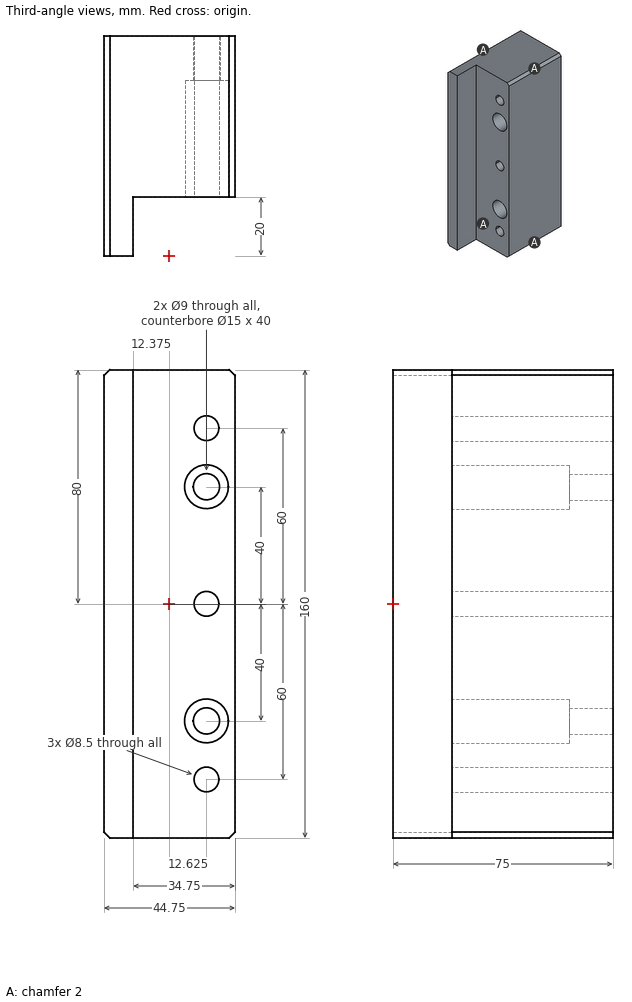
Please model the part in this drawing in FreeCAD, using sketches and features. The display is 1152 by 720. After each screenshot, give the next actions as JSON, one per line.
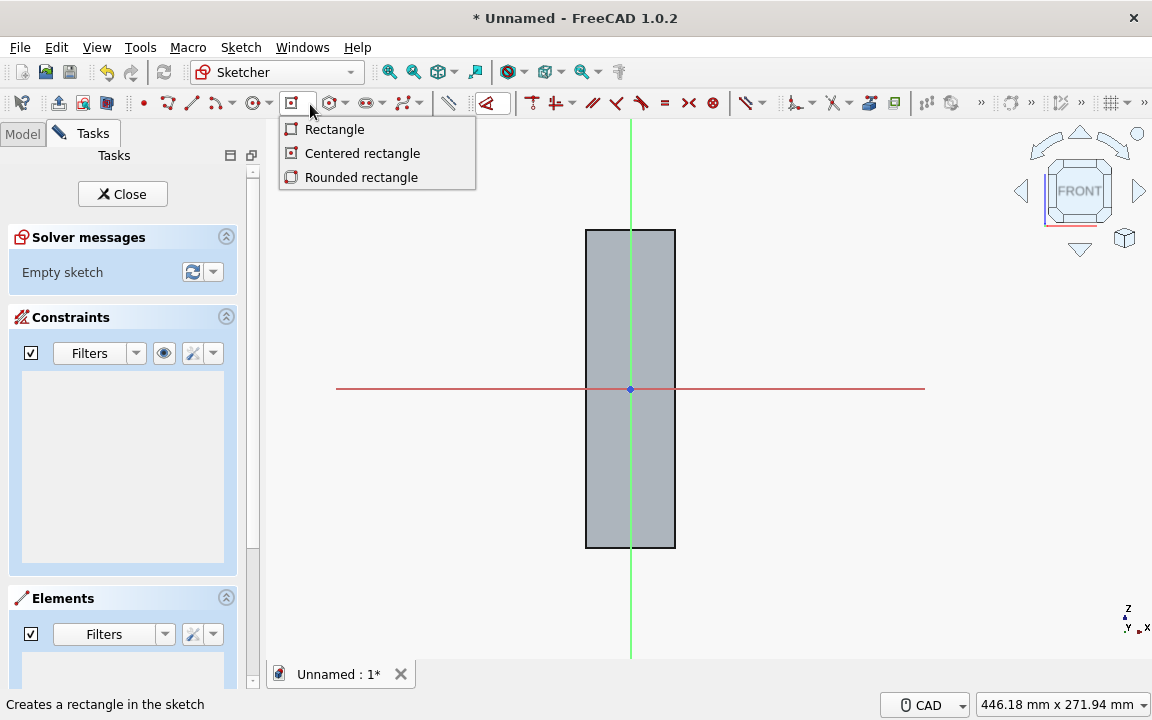
{"action": "left_click", "coordinate": [378, 129]}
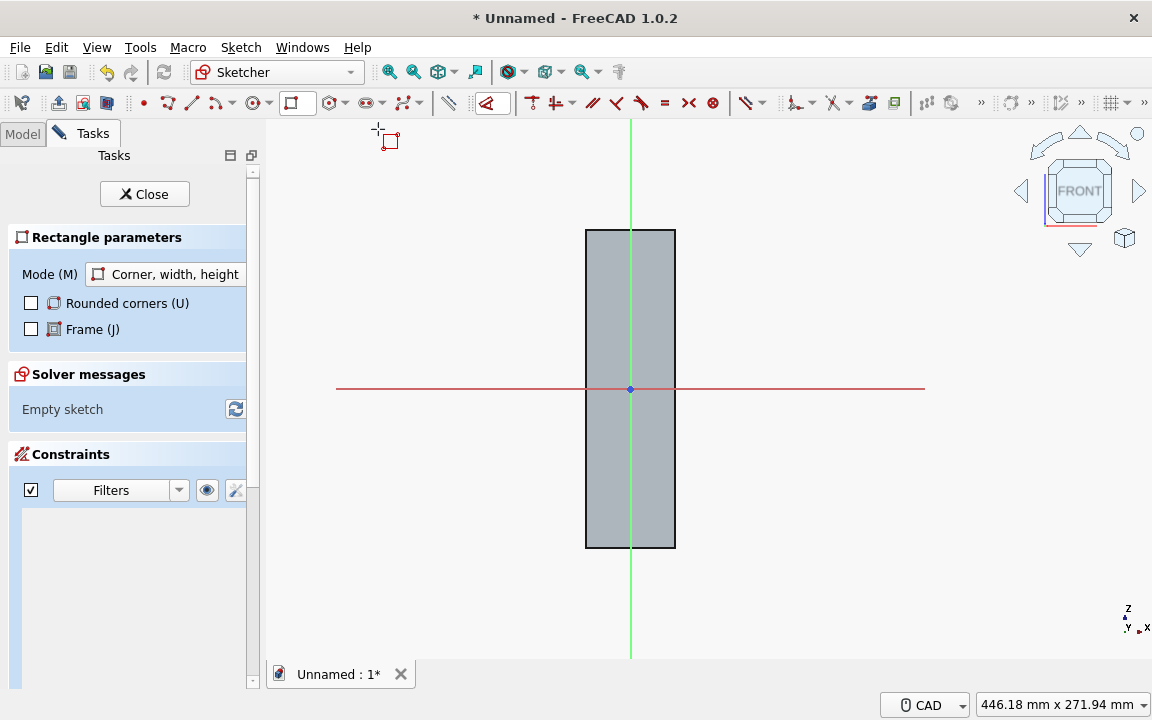
{"action": "left_click", "coordinate": [606, 230]}
{"action": "left_click", "coordinate": [675, 548]}
{"action": "key", "text": "Escape"}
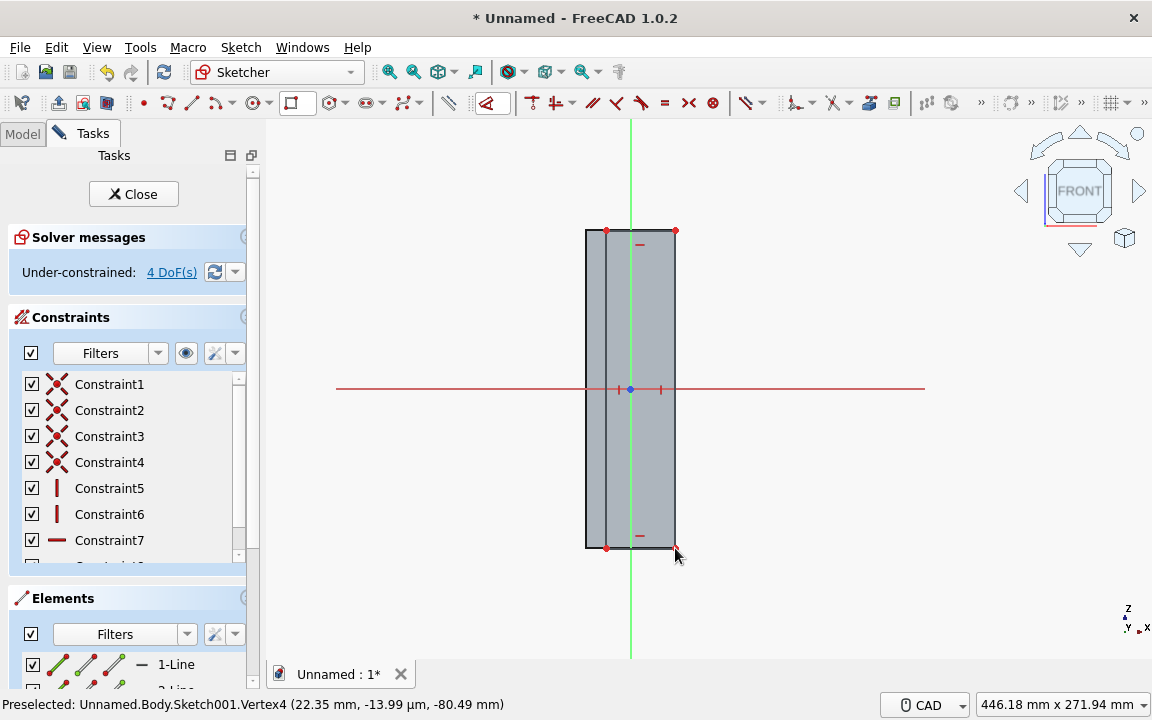
{"action": "key", "text": "d"}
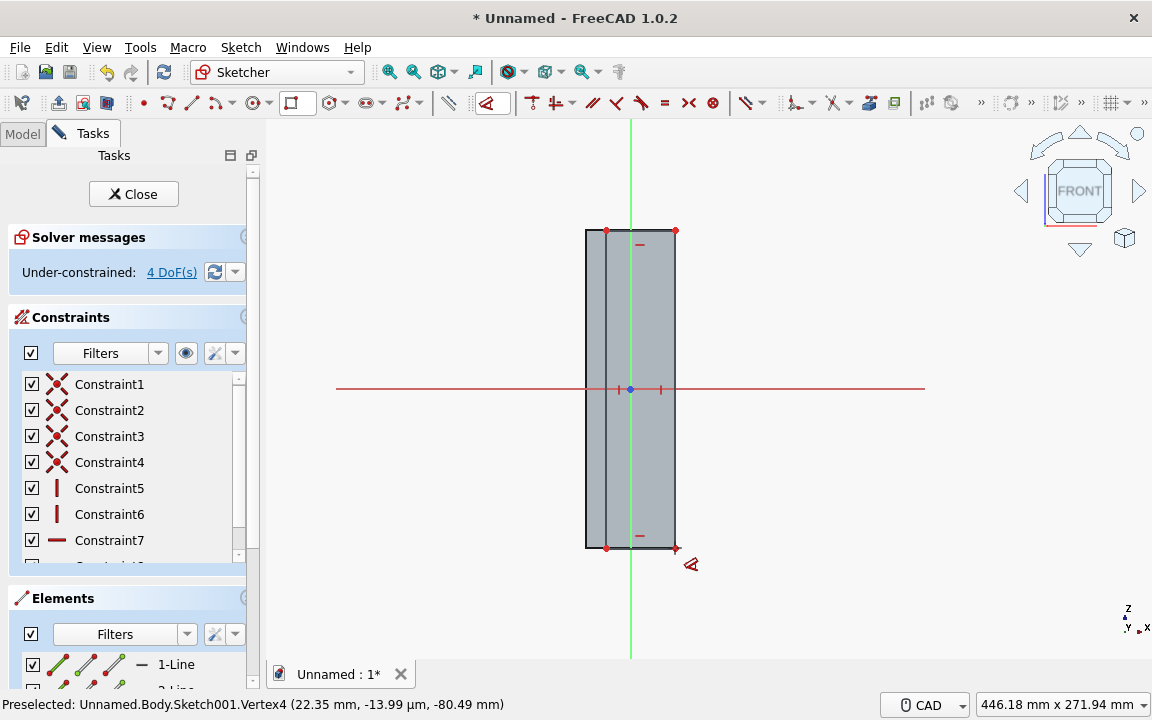
{"action": "left_click", "coordinate": [606, 326]}
{"action": "left_click", "coordinate": [572, 317]}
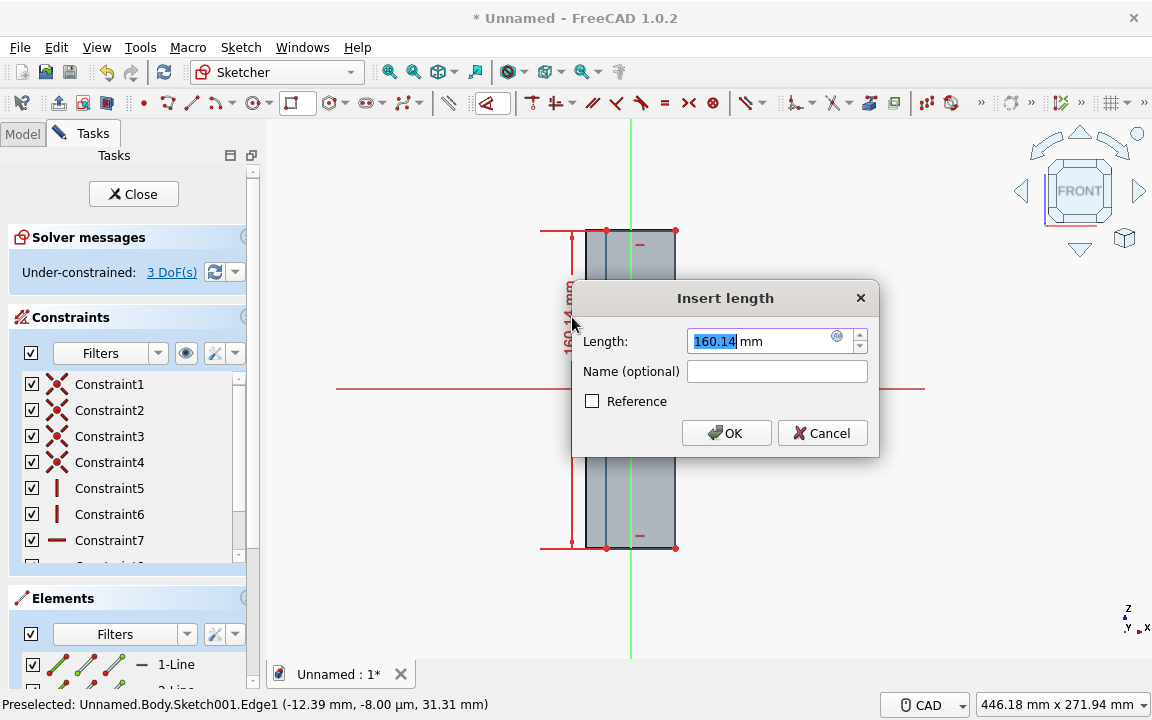
{"action": "type", "text": "160"}
{"action": "key", "text": "Return"}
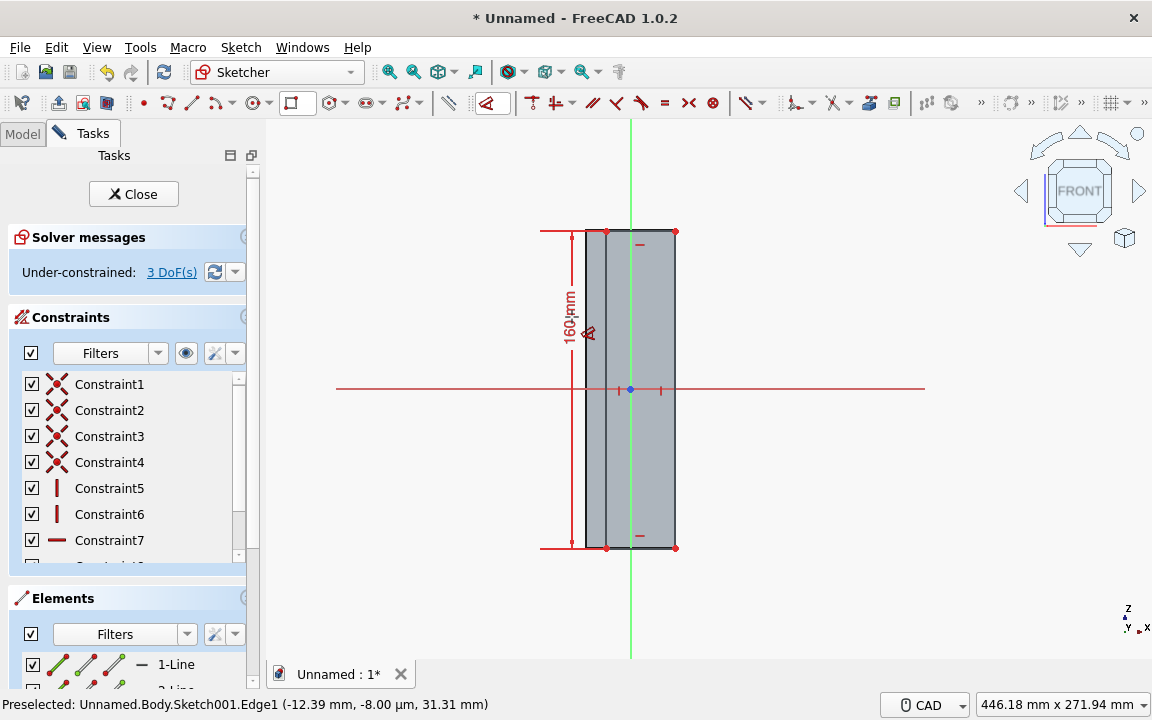
{"action": "left_click", "coordinate": [606, 231]}
{"action": "left_click", "coordinate": [572, 274]}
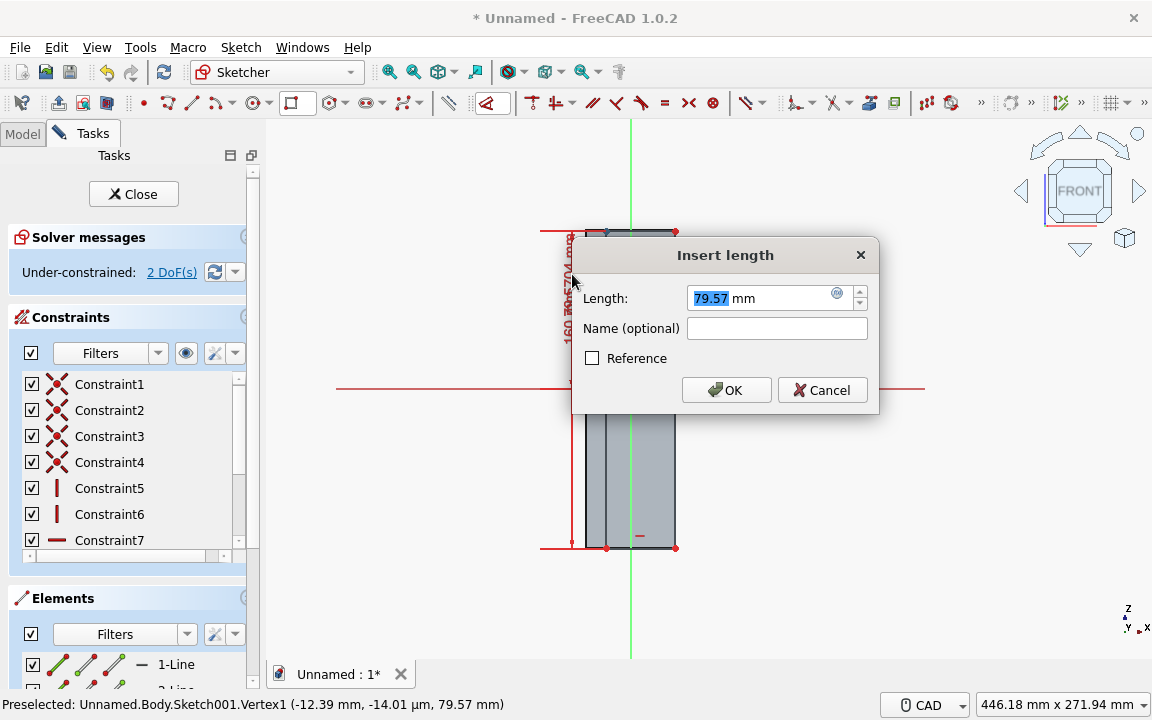
{"action": "type", "text": "80"}
{"action": "key", "text": "Return"}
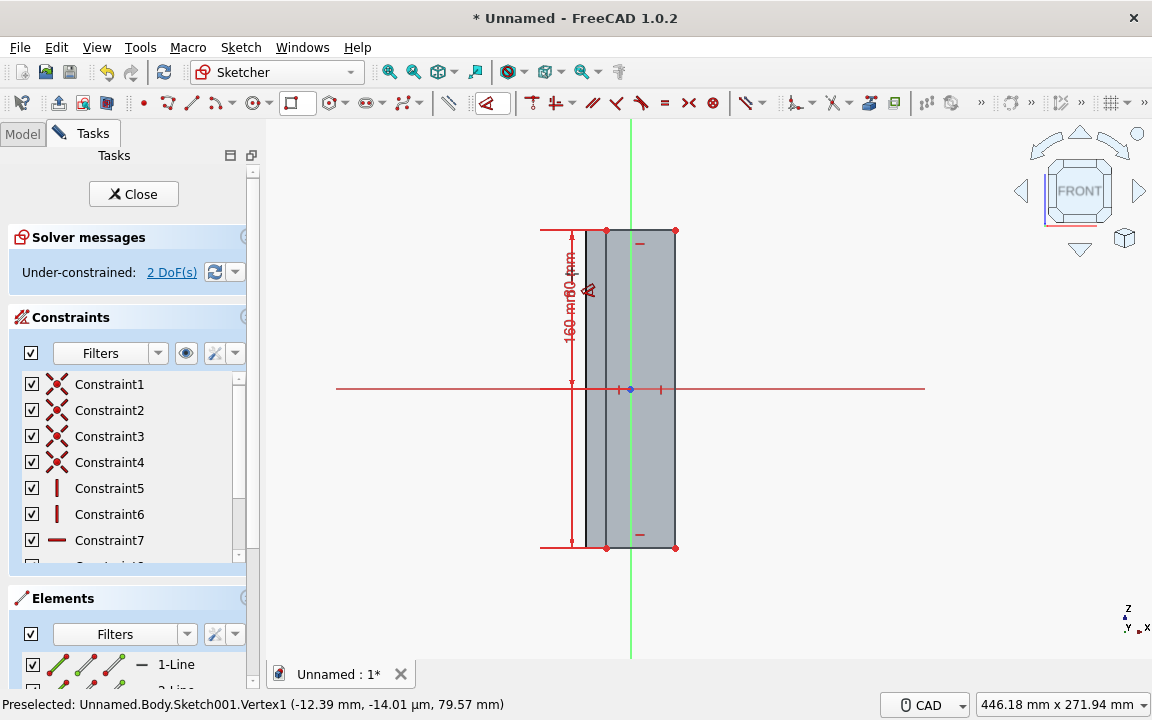
{"action": "left_click", "coordinate": [627, 548]}
{"action": "left_click", "coordinate": [656, 582]}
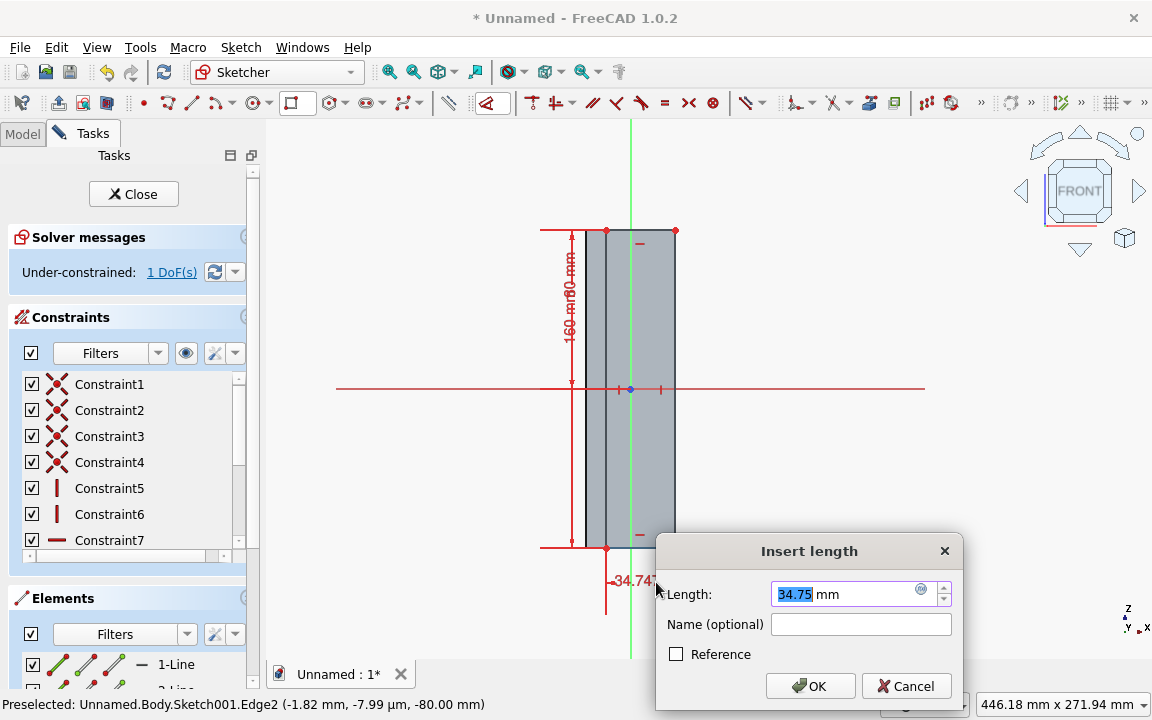
{"action": "type", "text": "34.75"}
{"action": "key", "text": "Return"}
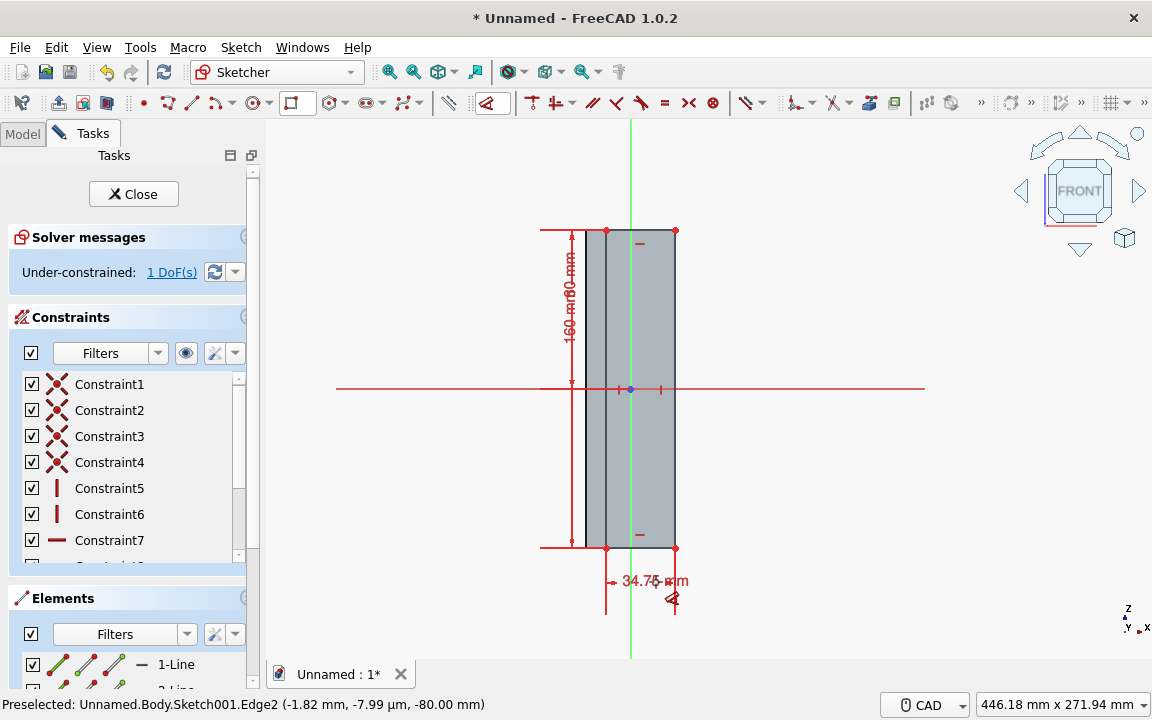
{"action": "scroll", "coordinate": [606, 230], "scroll_direction": "up", "scroll_amount": 3}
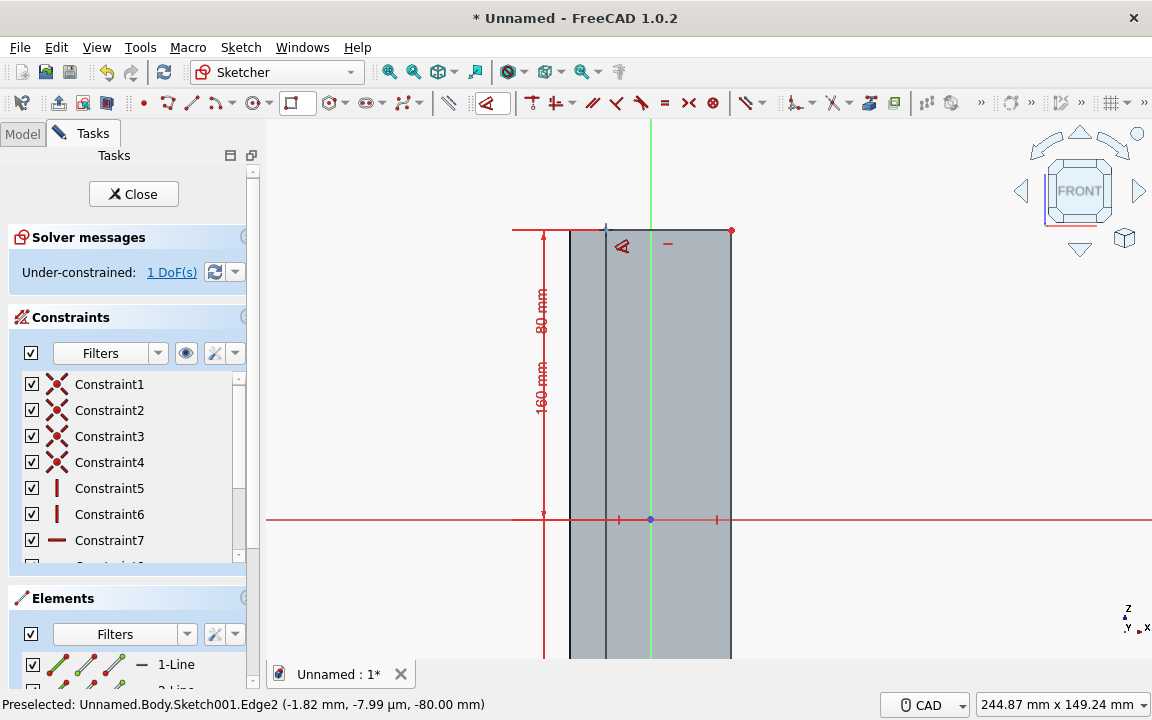
{"action": "left_click", "coordinate": [606, 230]}
{"action": "left_click", "coordinate": [628, 196]}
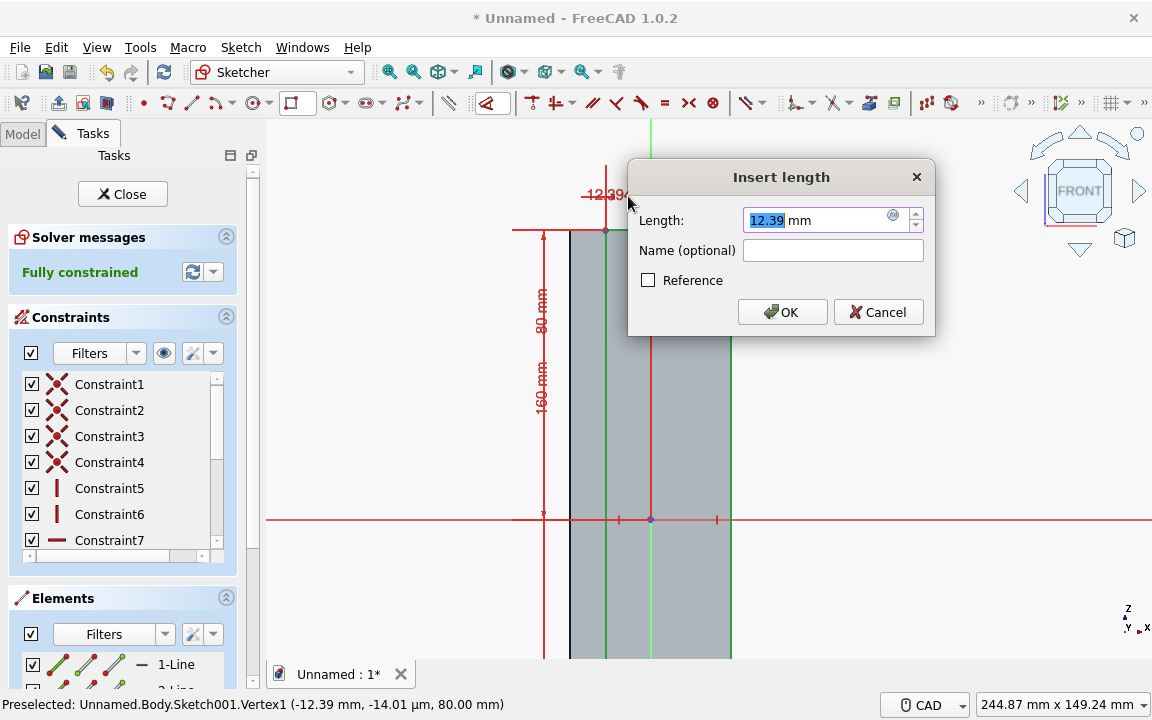
{"action": "type", "text": "12.375"}
{"action": "key", "text": "Return"}
{"action": "key", "text": "Escape"}